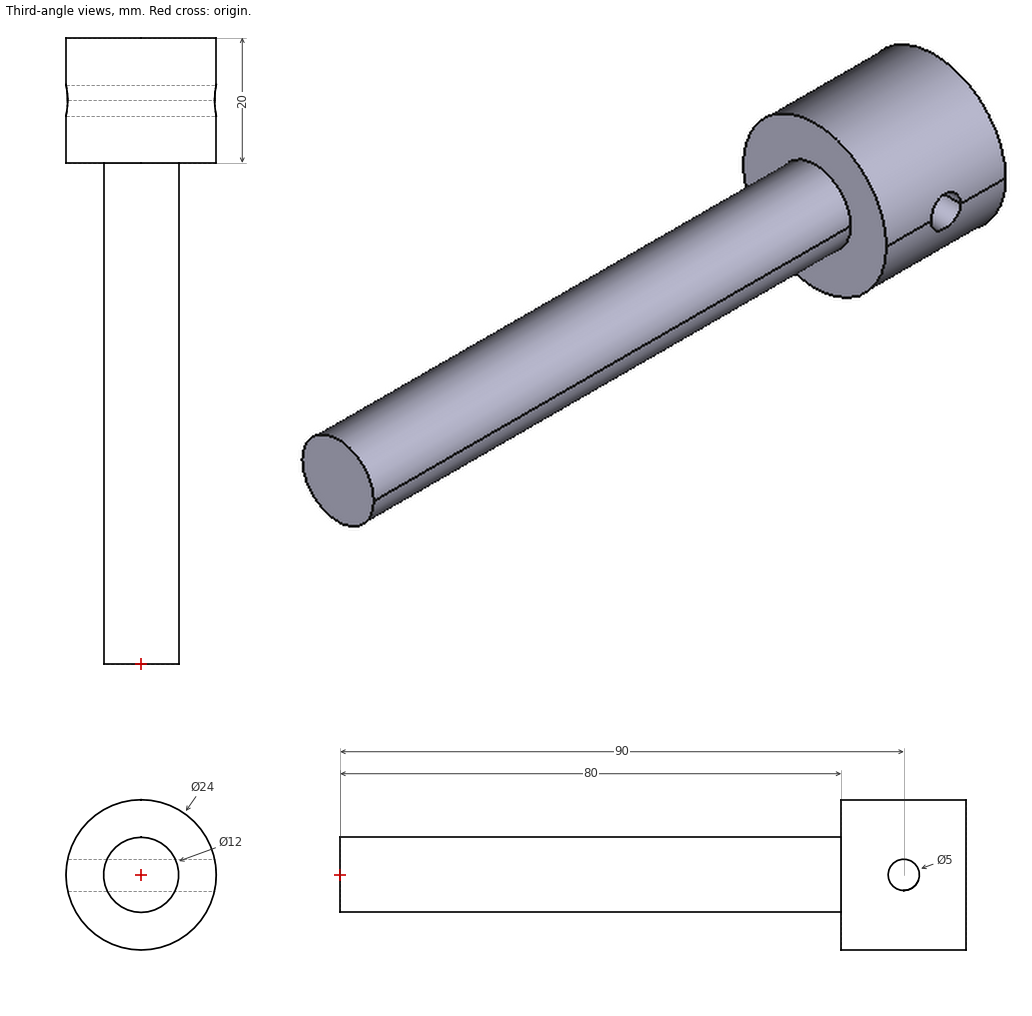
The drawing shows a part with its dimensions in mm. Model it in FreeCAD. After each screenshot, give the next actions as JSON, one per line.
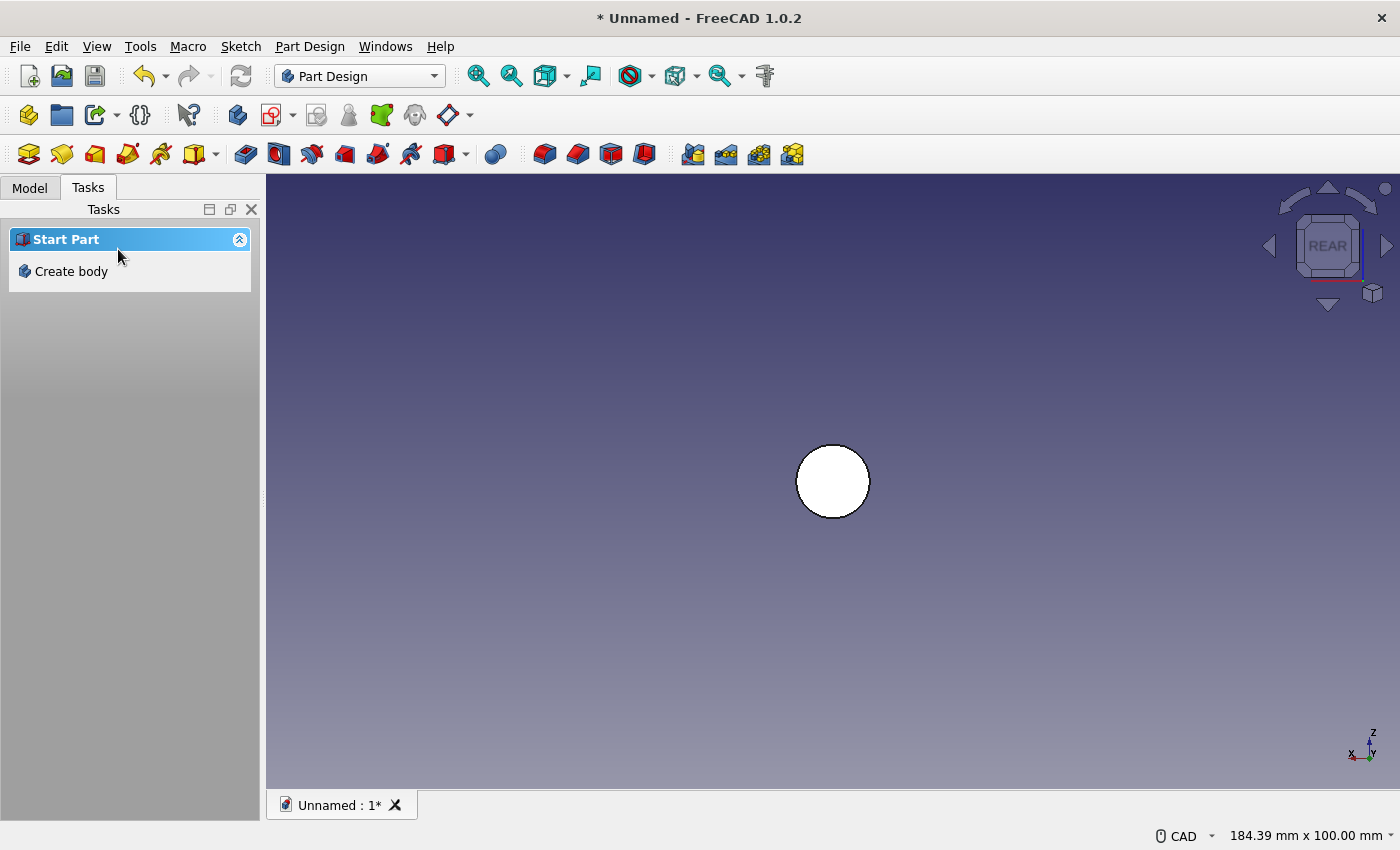
{"action": "key", "text": "v f"}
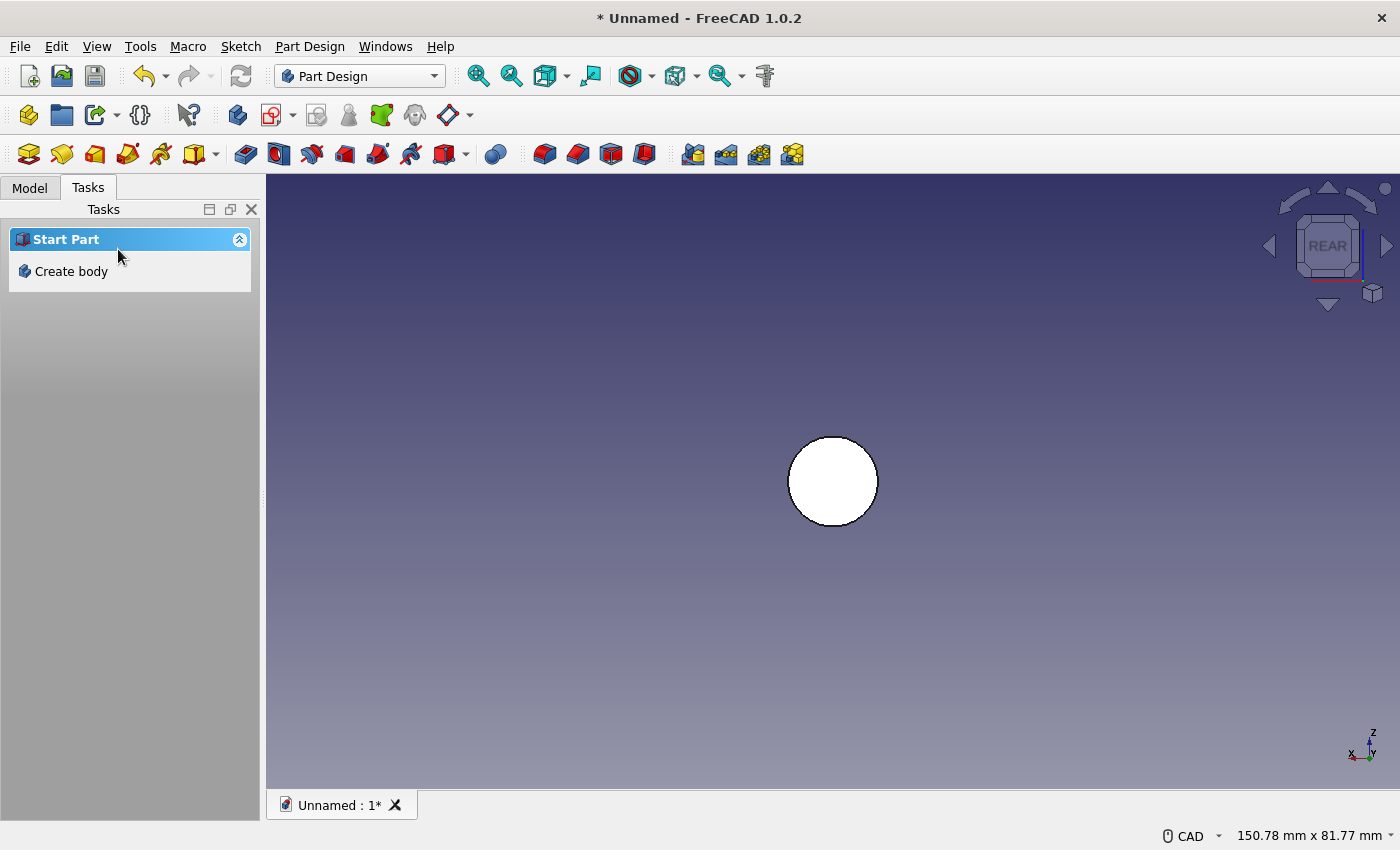
{"action": "left_click", "coordinate": [833, 481]}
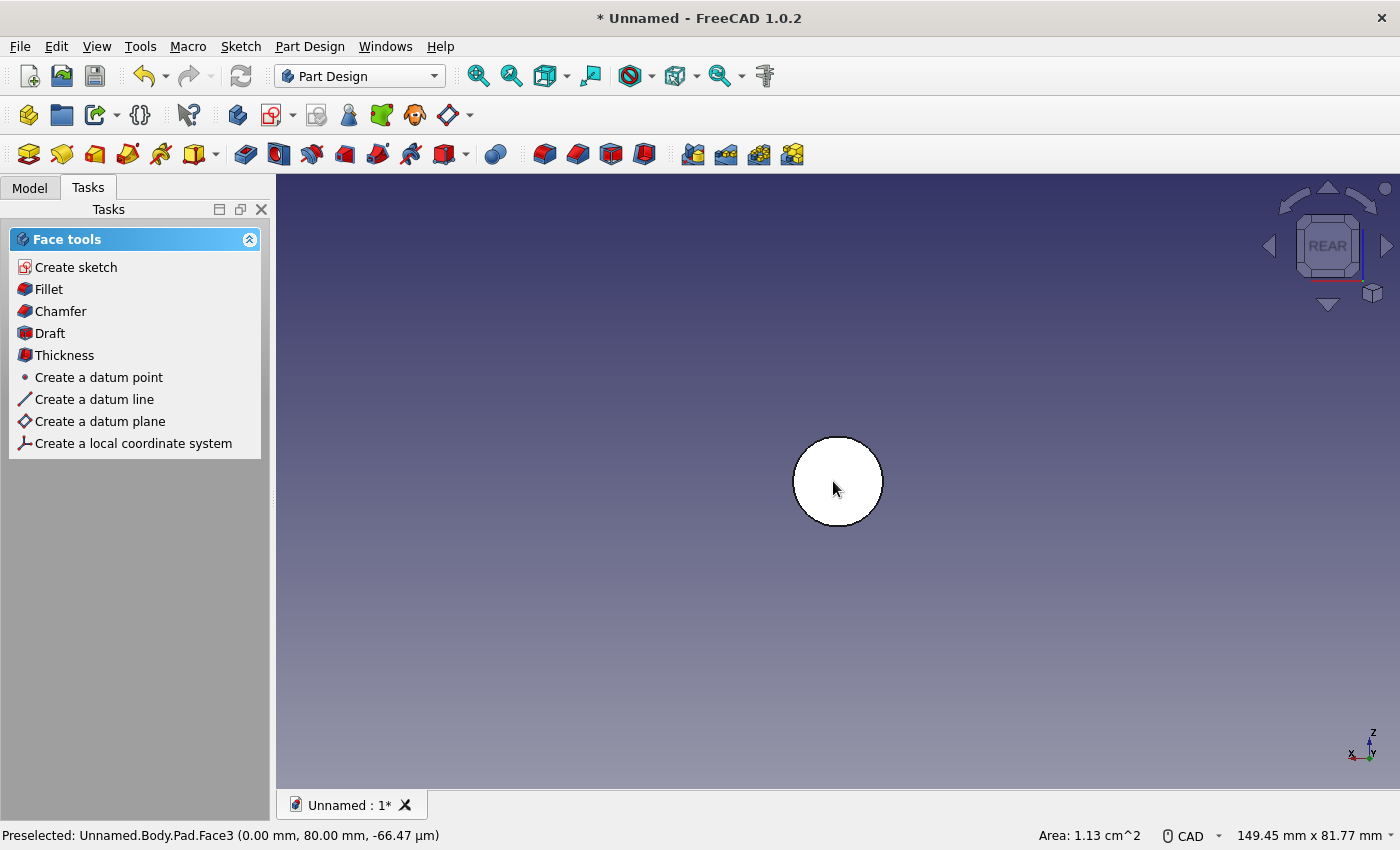
{"action": "left_click", "coordinate": [270, 116]}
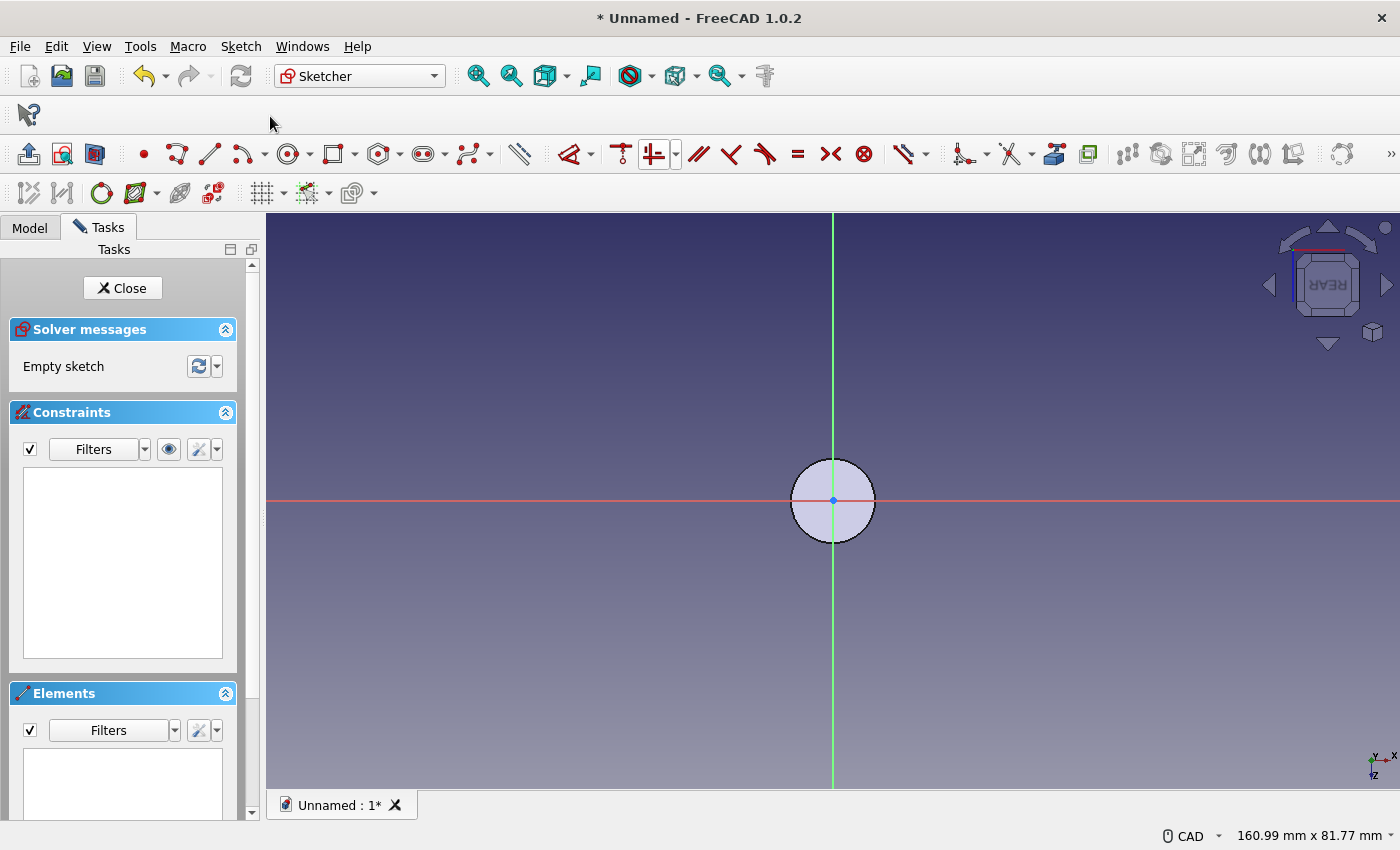
{"action": "scroll", "coordinate": [889, 501], "scroll_direction": "up", "scroll_amount": 4}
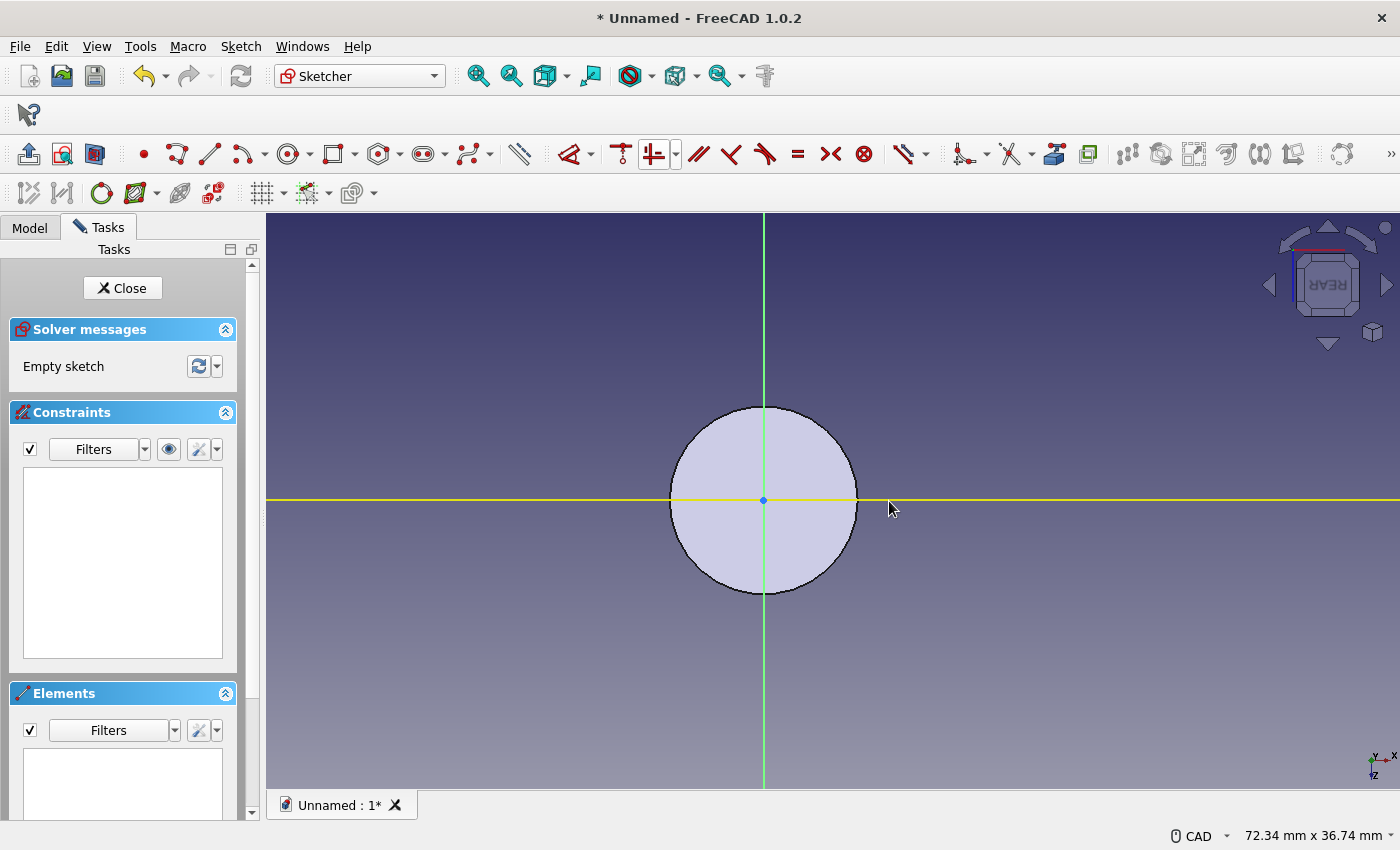
{"action": "left_click", "coordinate": [288, 154]}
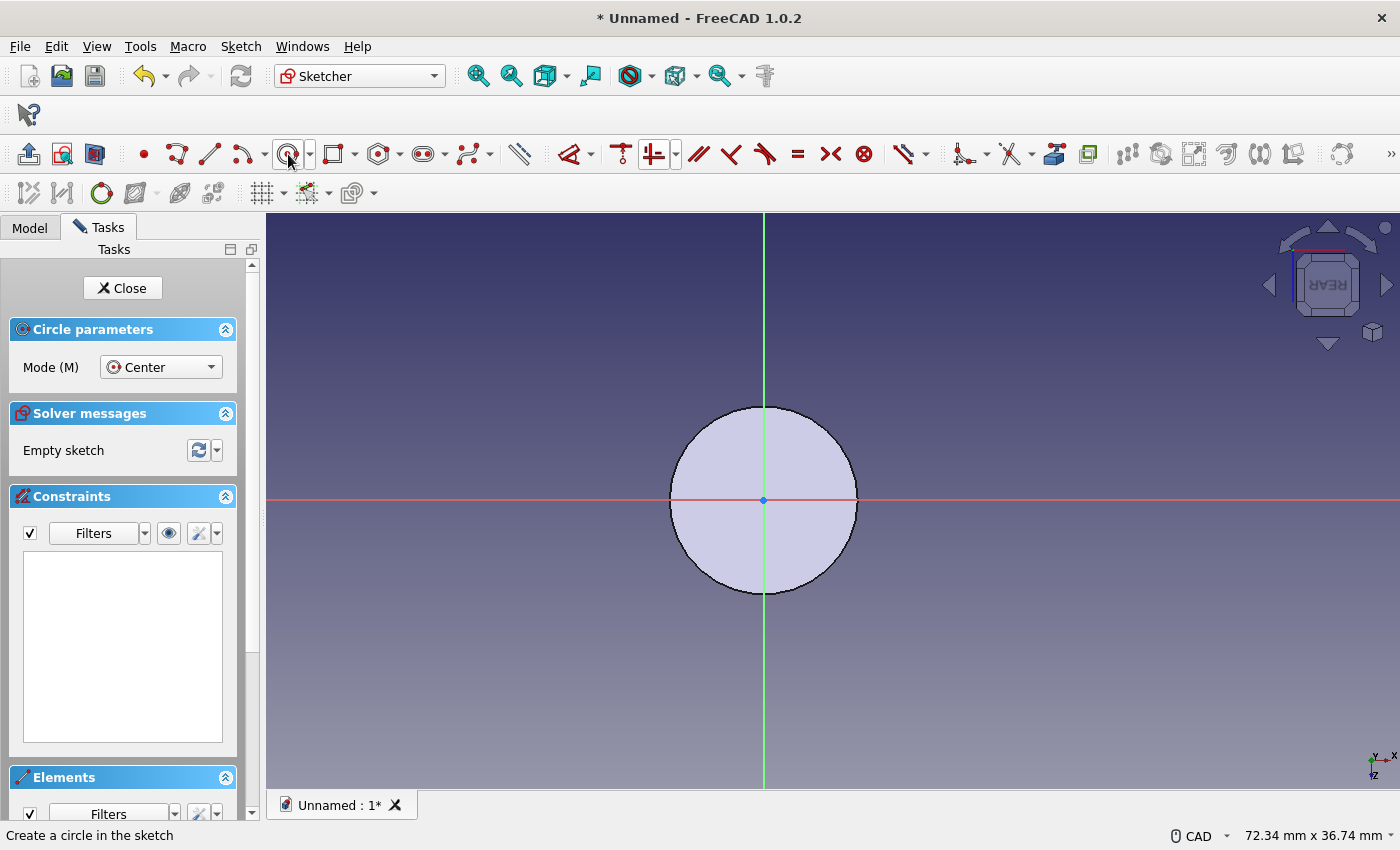
{"action": "left_click", "coordinate": [764, 500]}
{"action": "left_click", "coordinate": [897, 367]}
{"action": "key", "text": "Escape"}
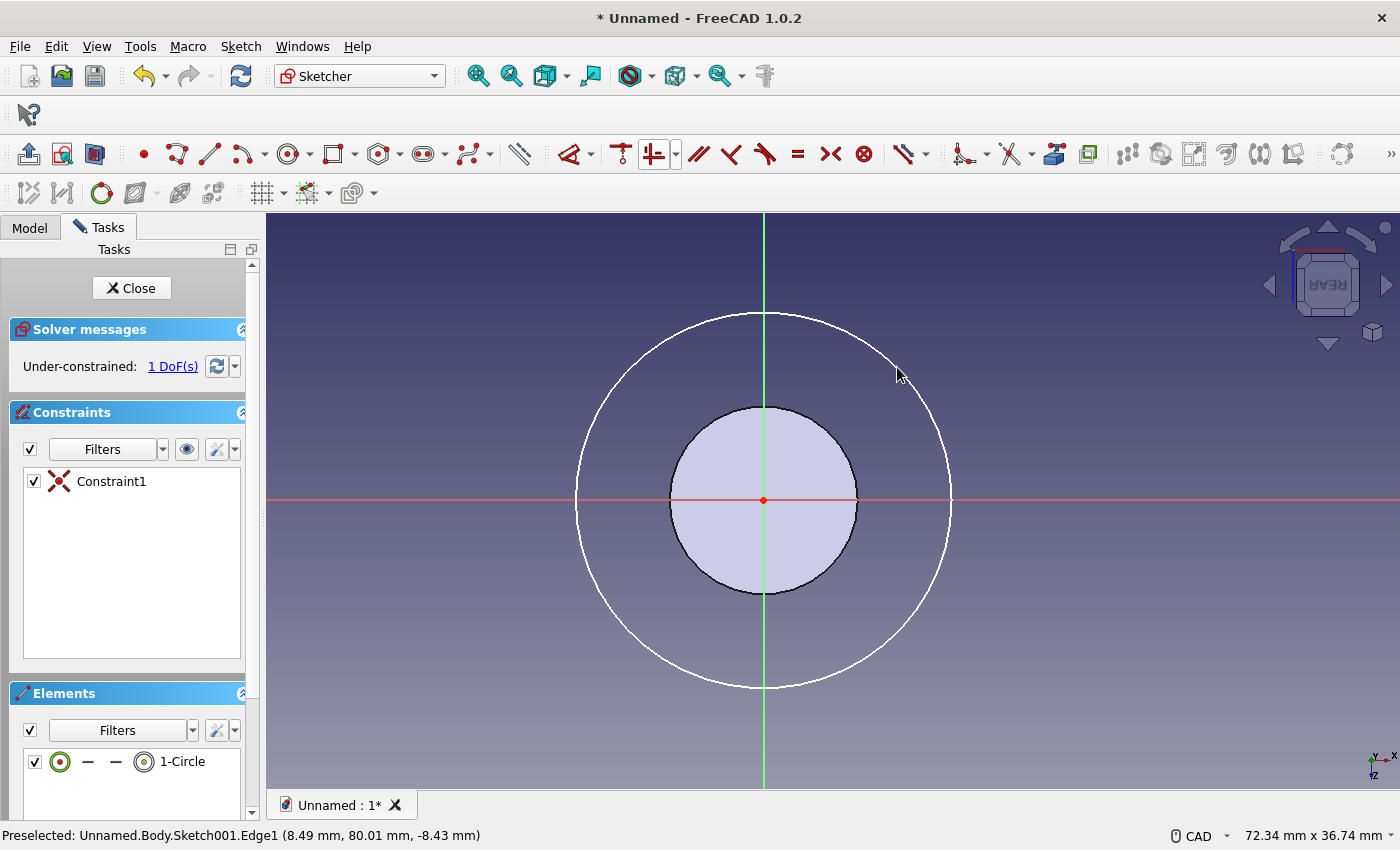
{"action": "left_click", "coordinate": [896, 367]}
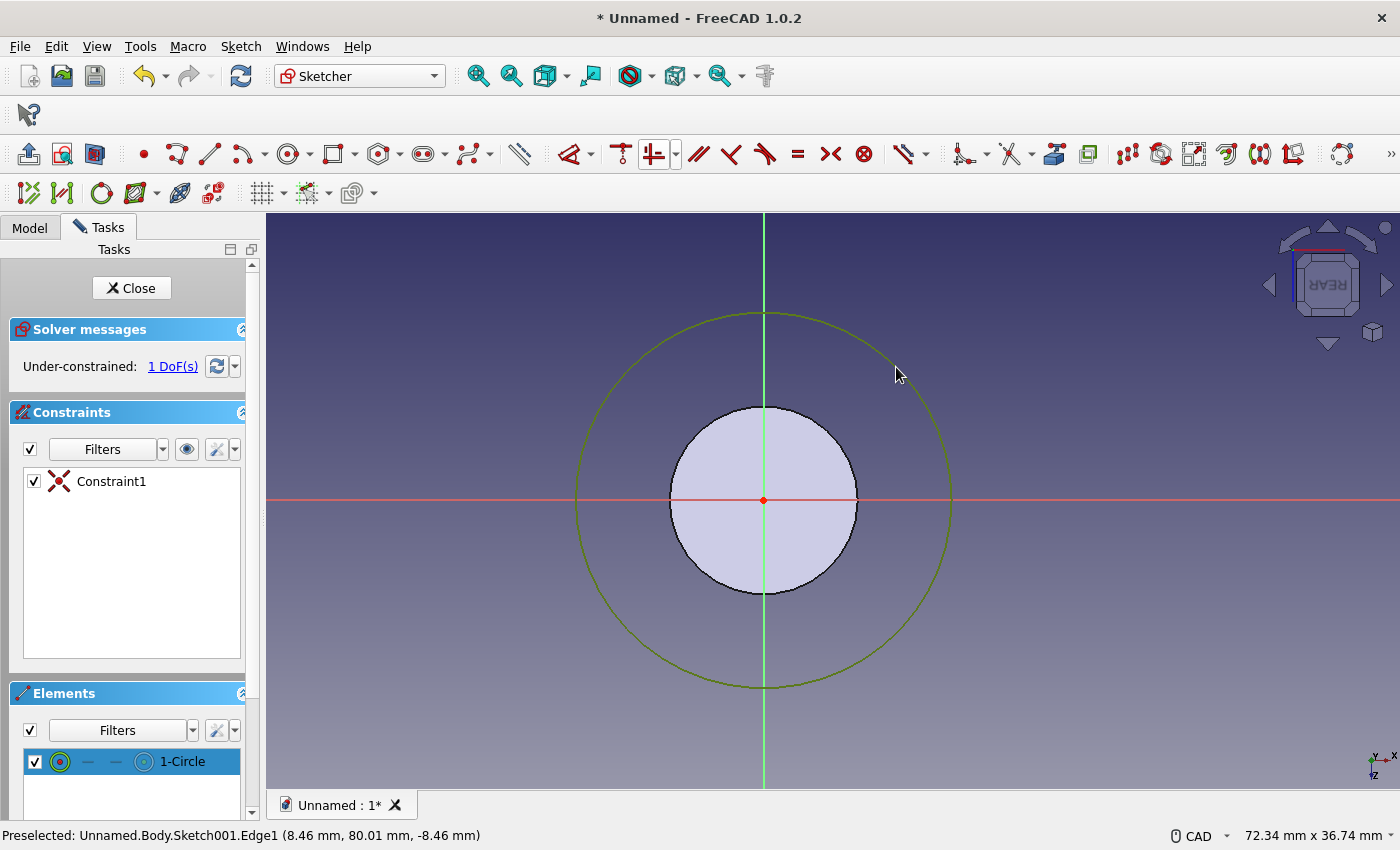
{"action": "key", "text": "k o"}